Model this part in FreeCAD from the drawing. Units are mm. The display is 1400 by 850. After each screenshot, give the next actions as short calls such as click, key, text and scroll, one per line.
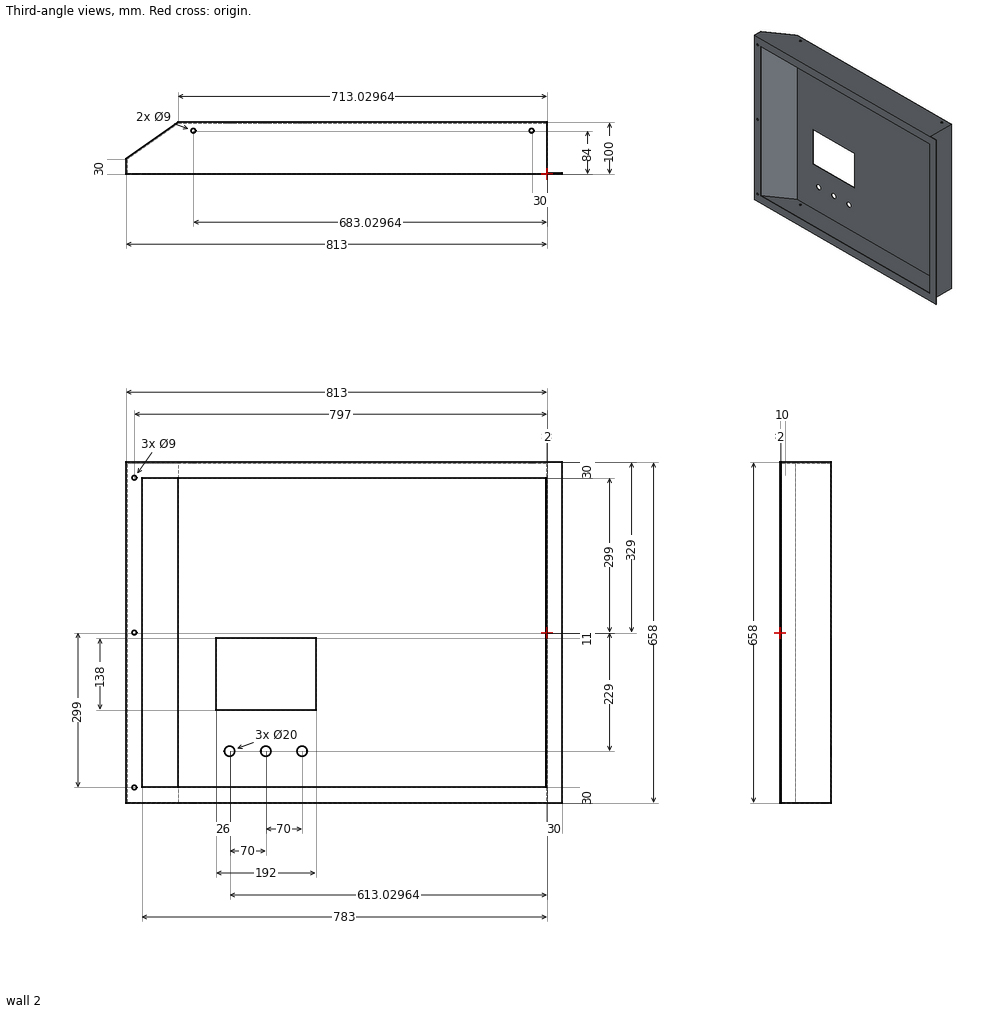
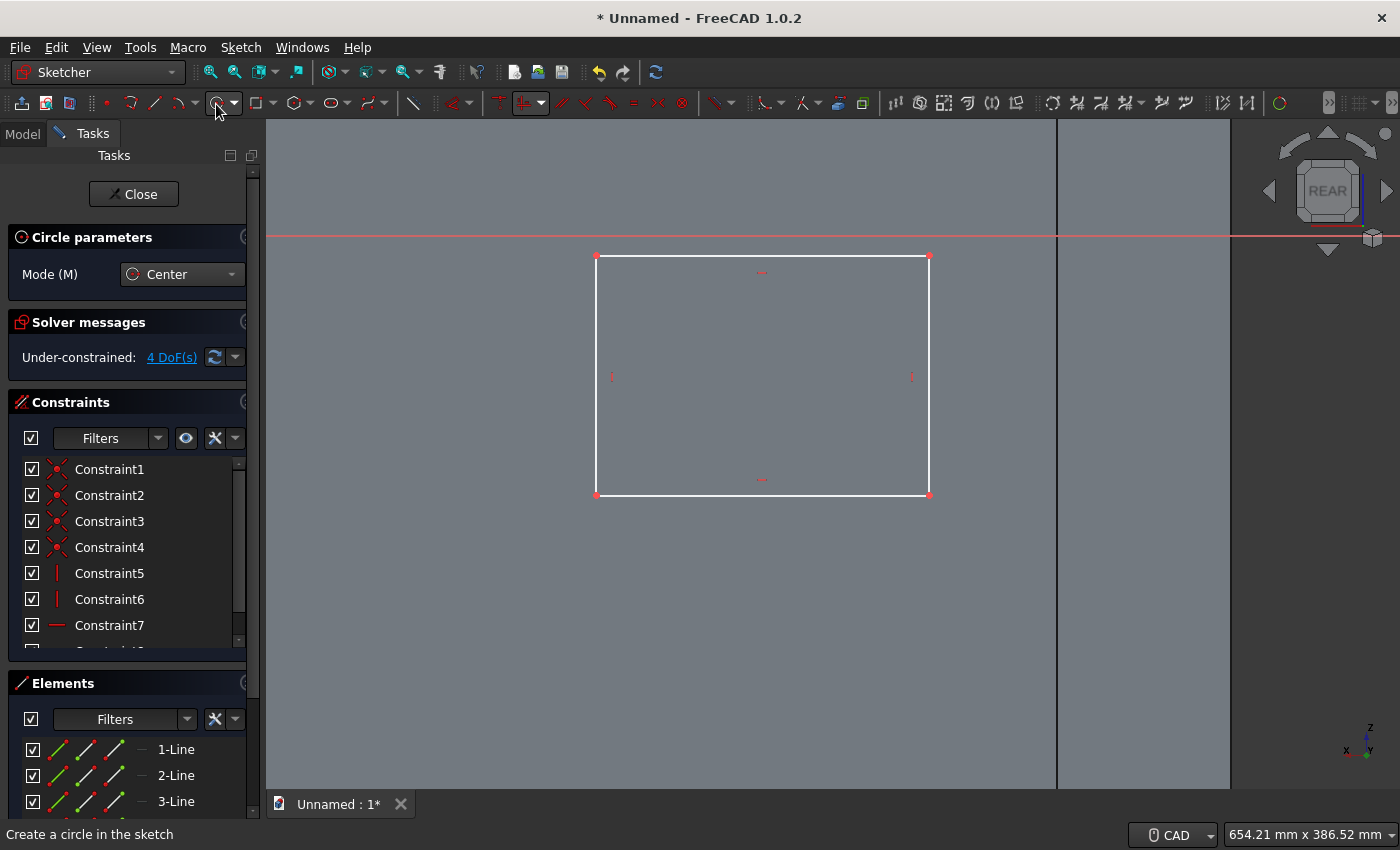
scroll(884, 633, up, 2)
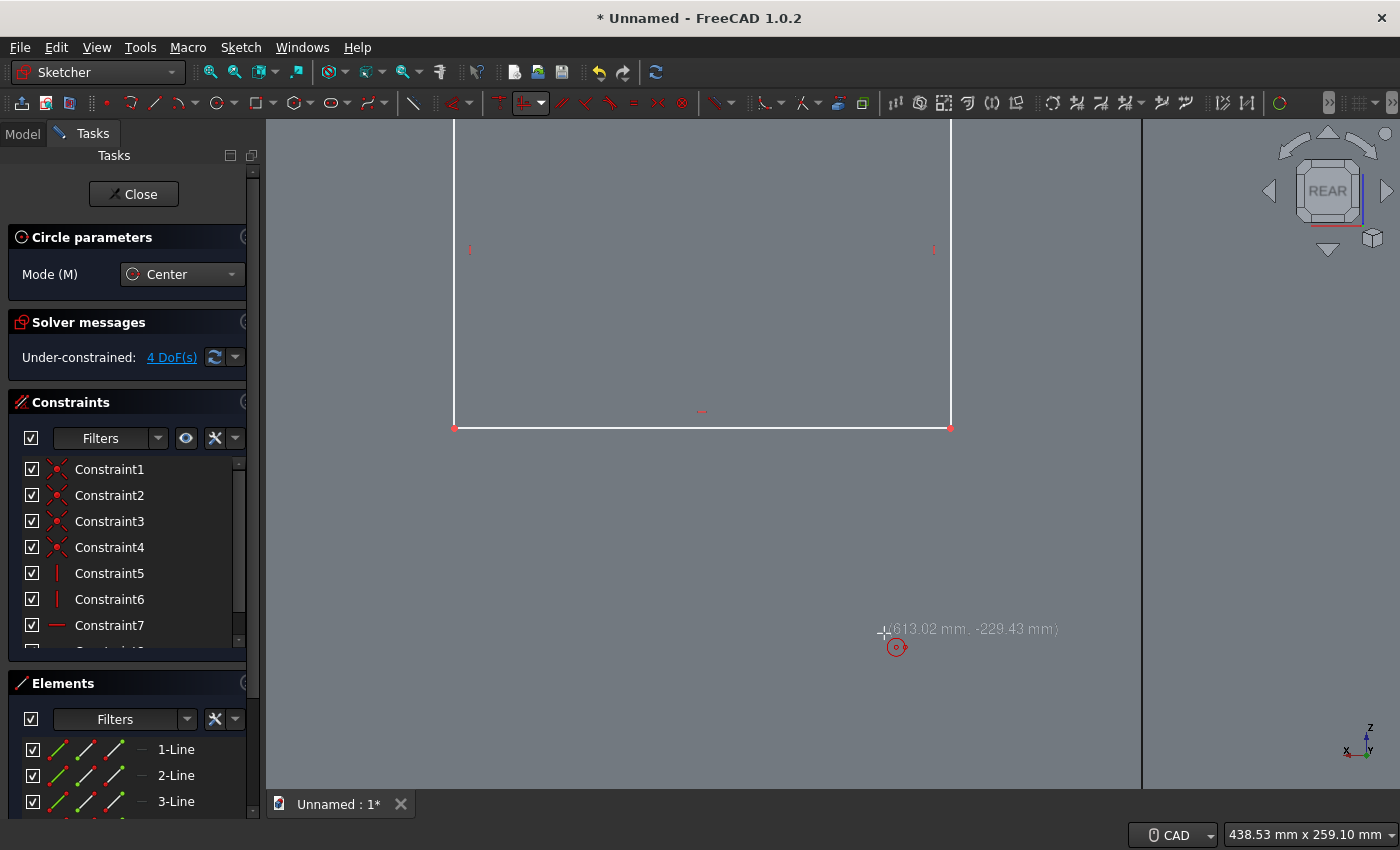
click(884, 633)
click(902, 615)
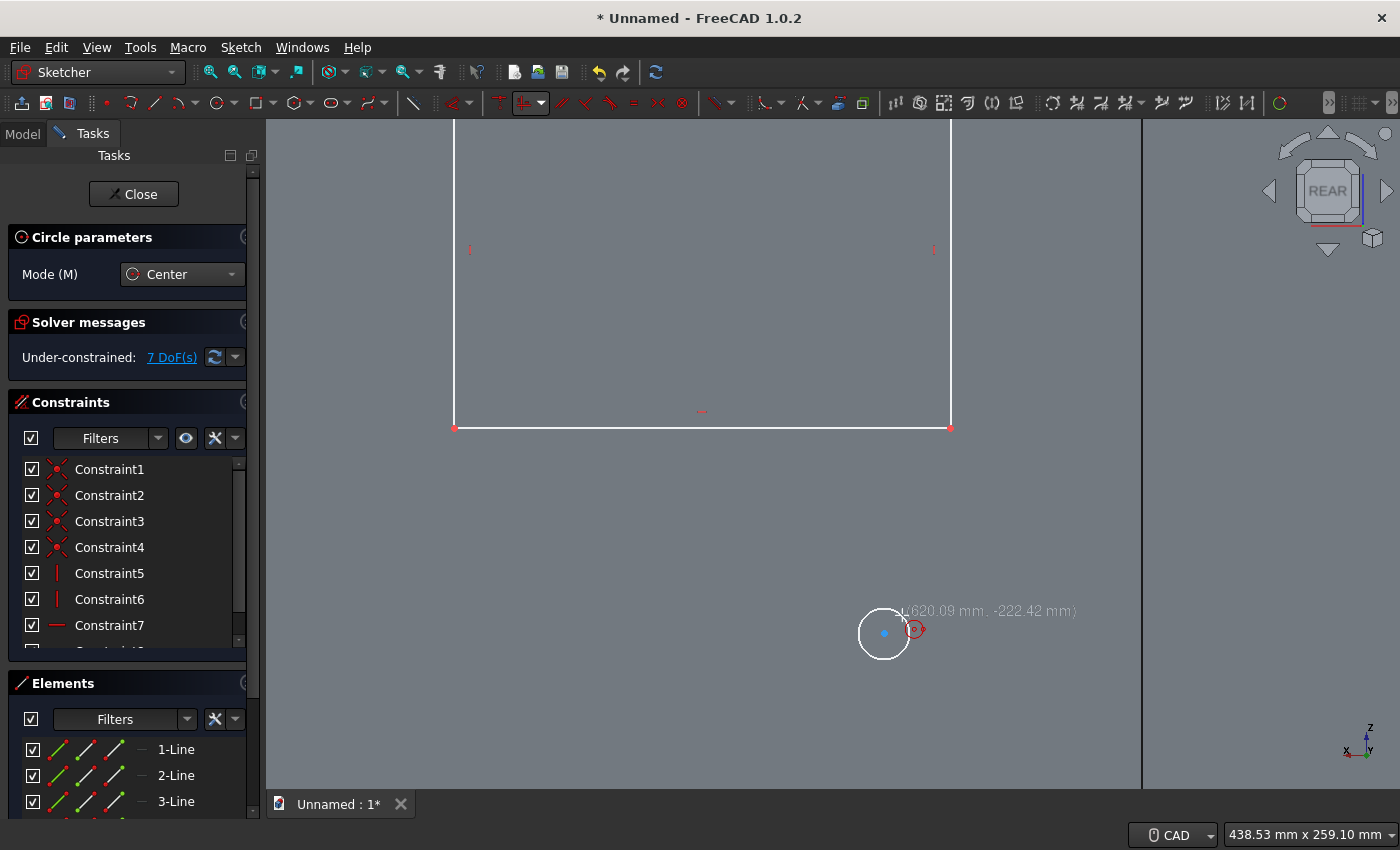
click(703, 633)
click(721, 615)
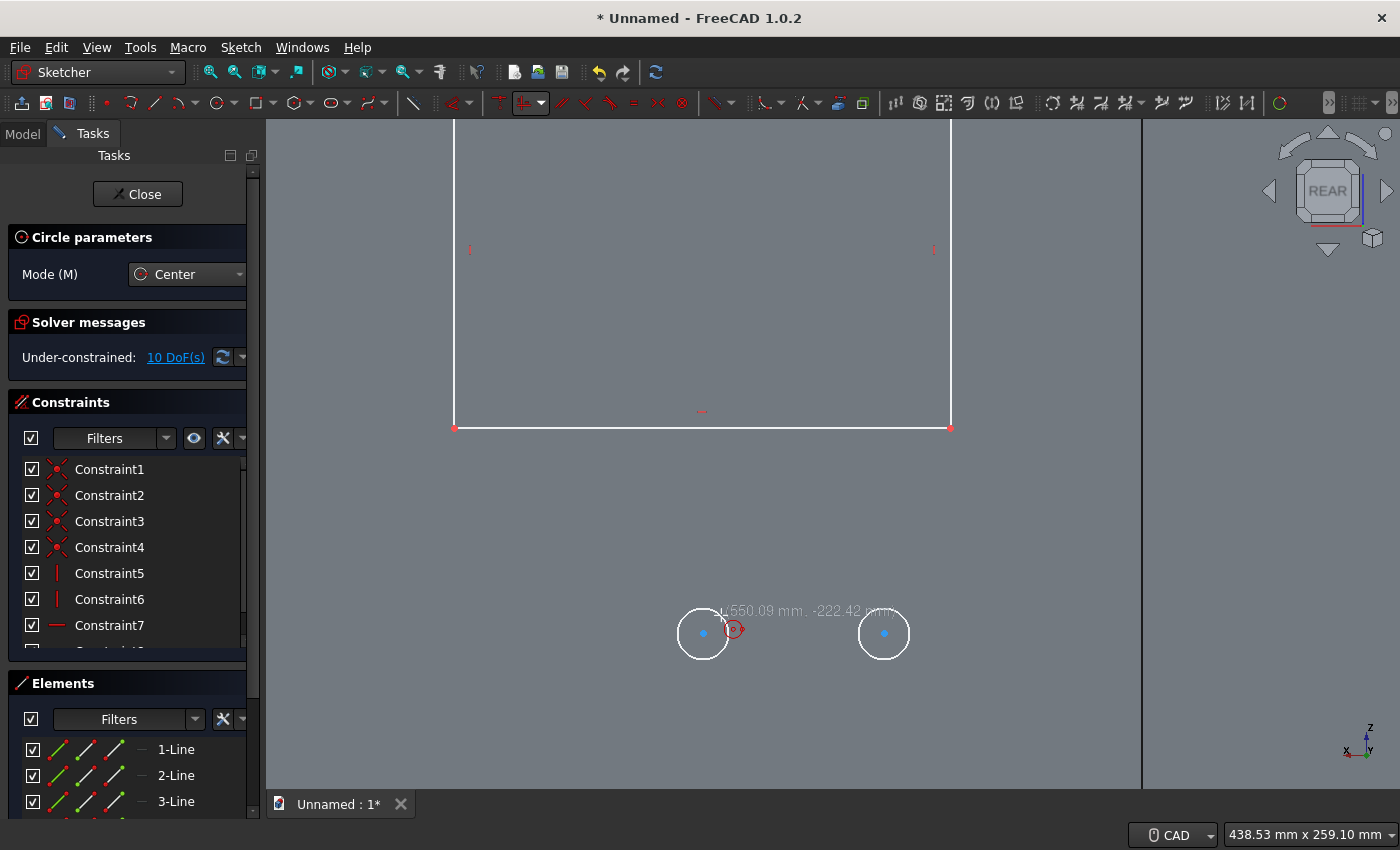
click(522, 633)
click(540, 615)
key(Escape)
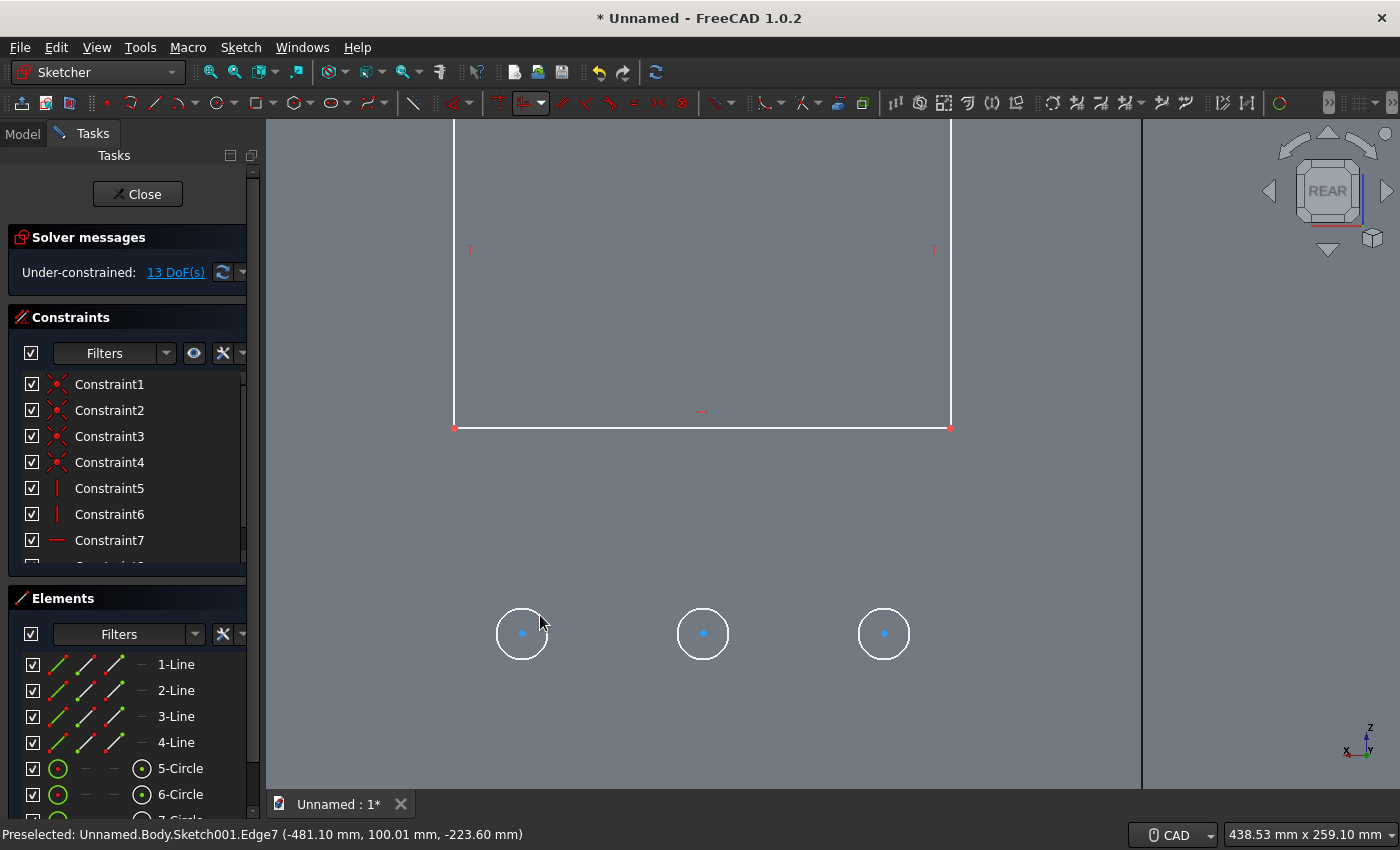
click(902, 616)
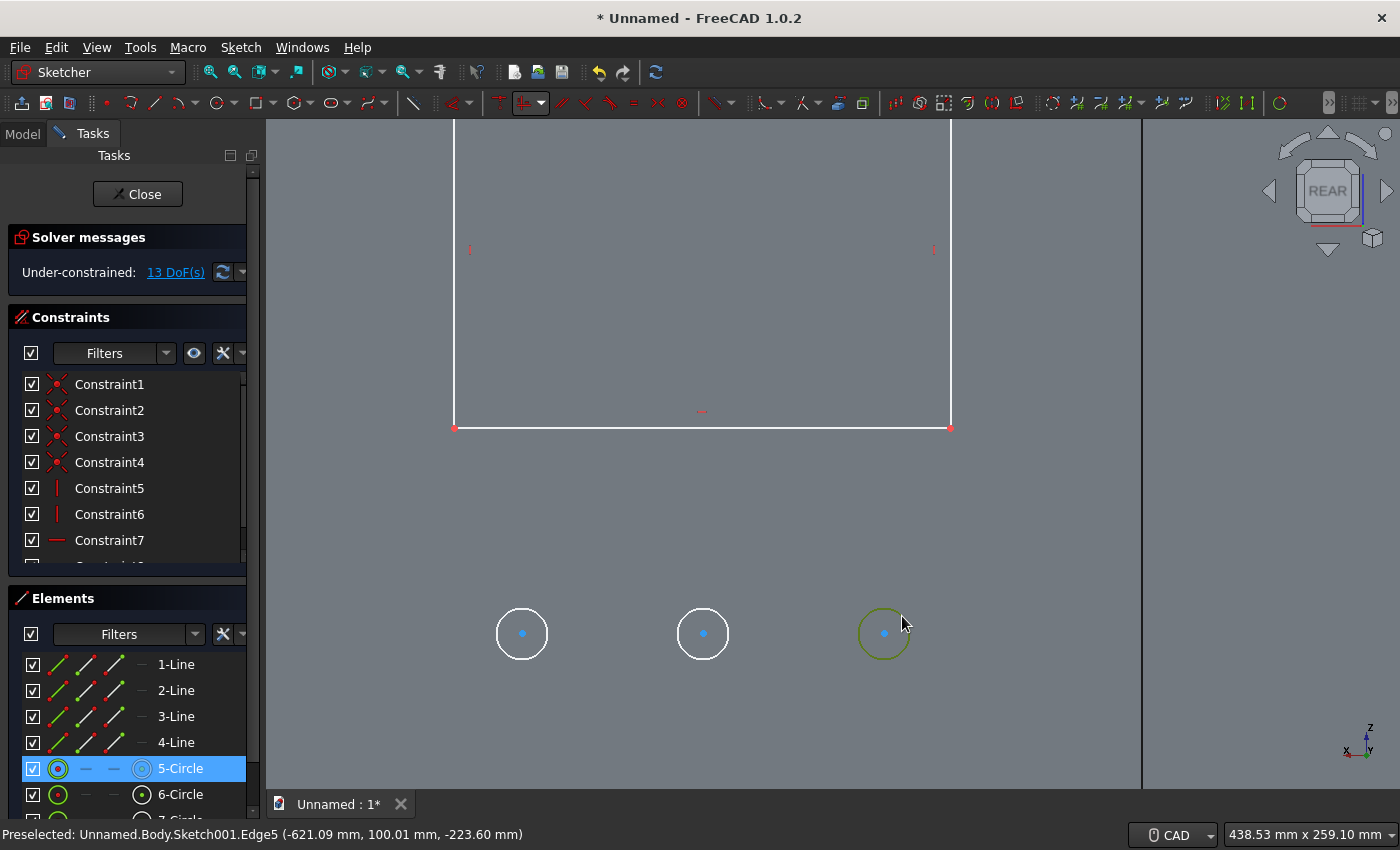
click(721, 616)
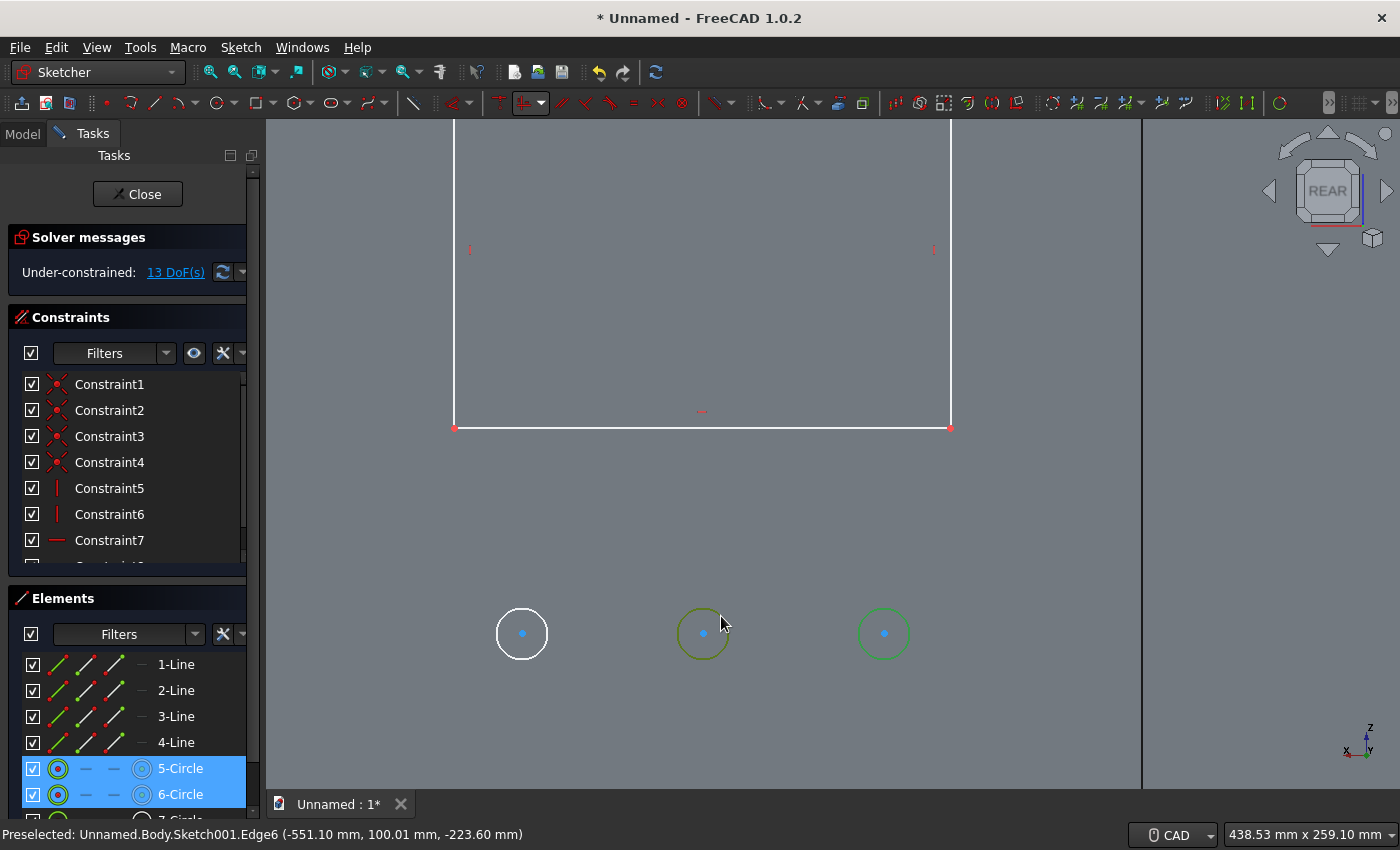
click(540, 616)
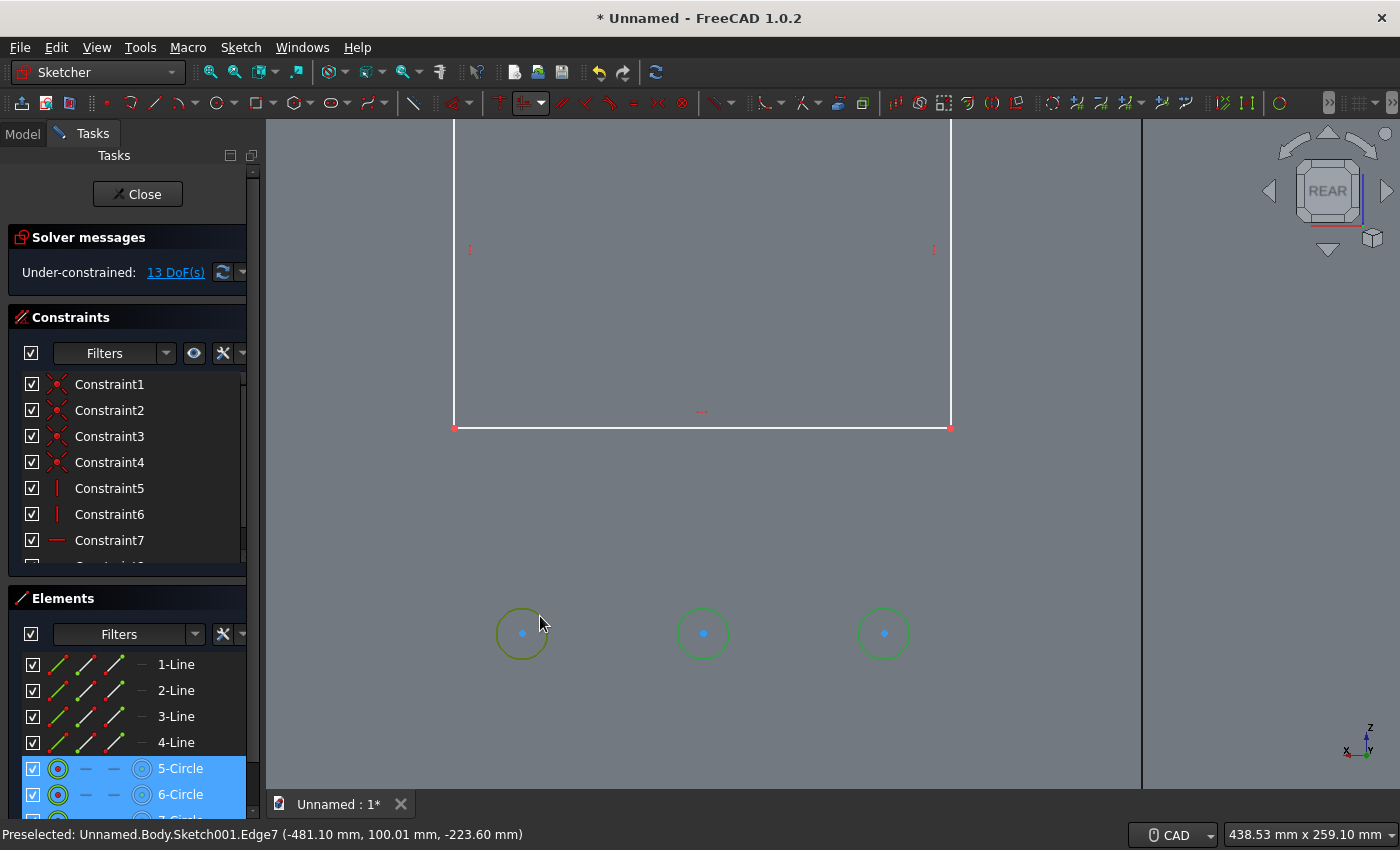
key(e)